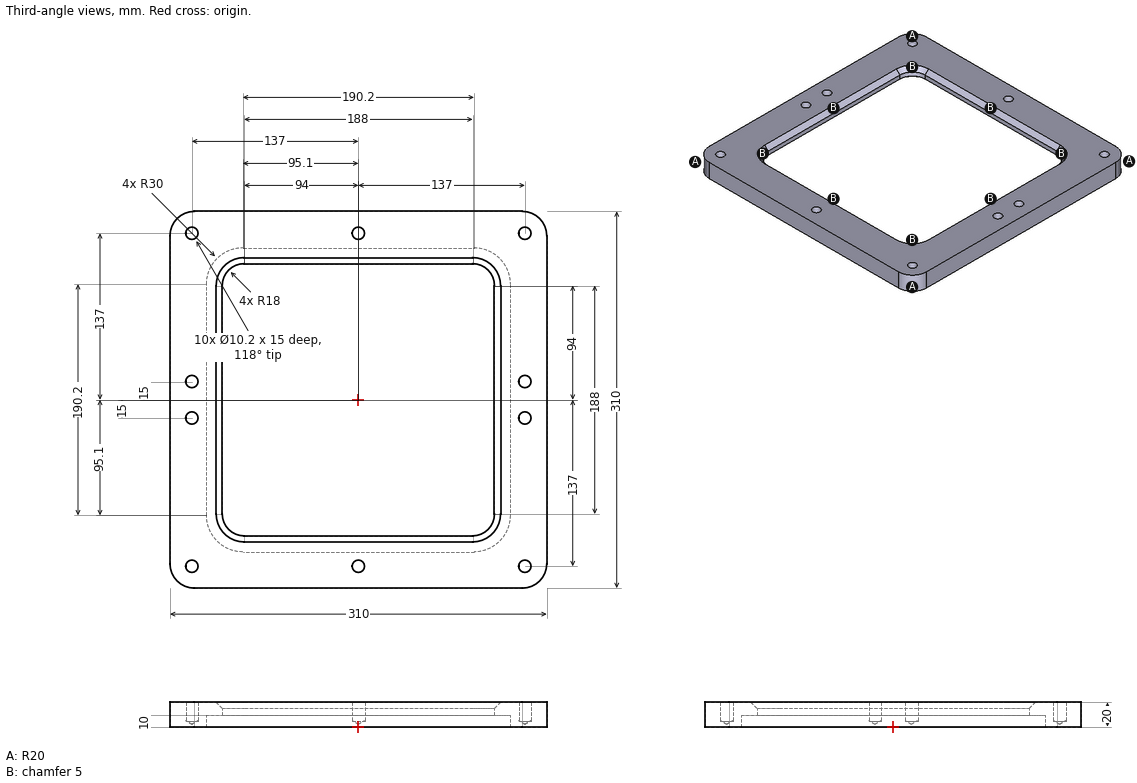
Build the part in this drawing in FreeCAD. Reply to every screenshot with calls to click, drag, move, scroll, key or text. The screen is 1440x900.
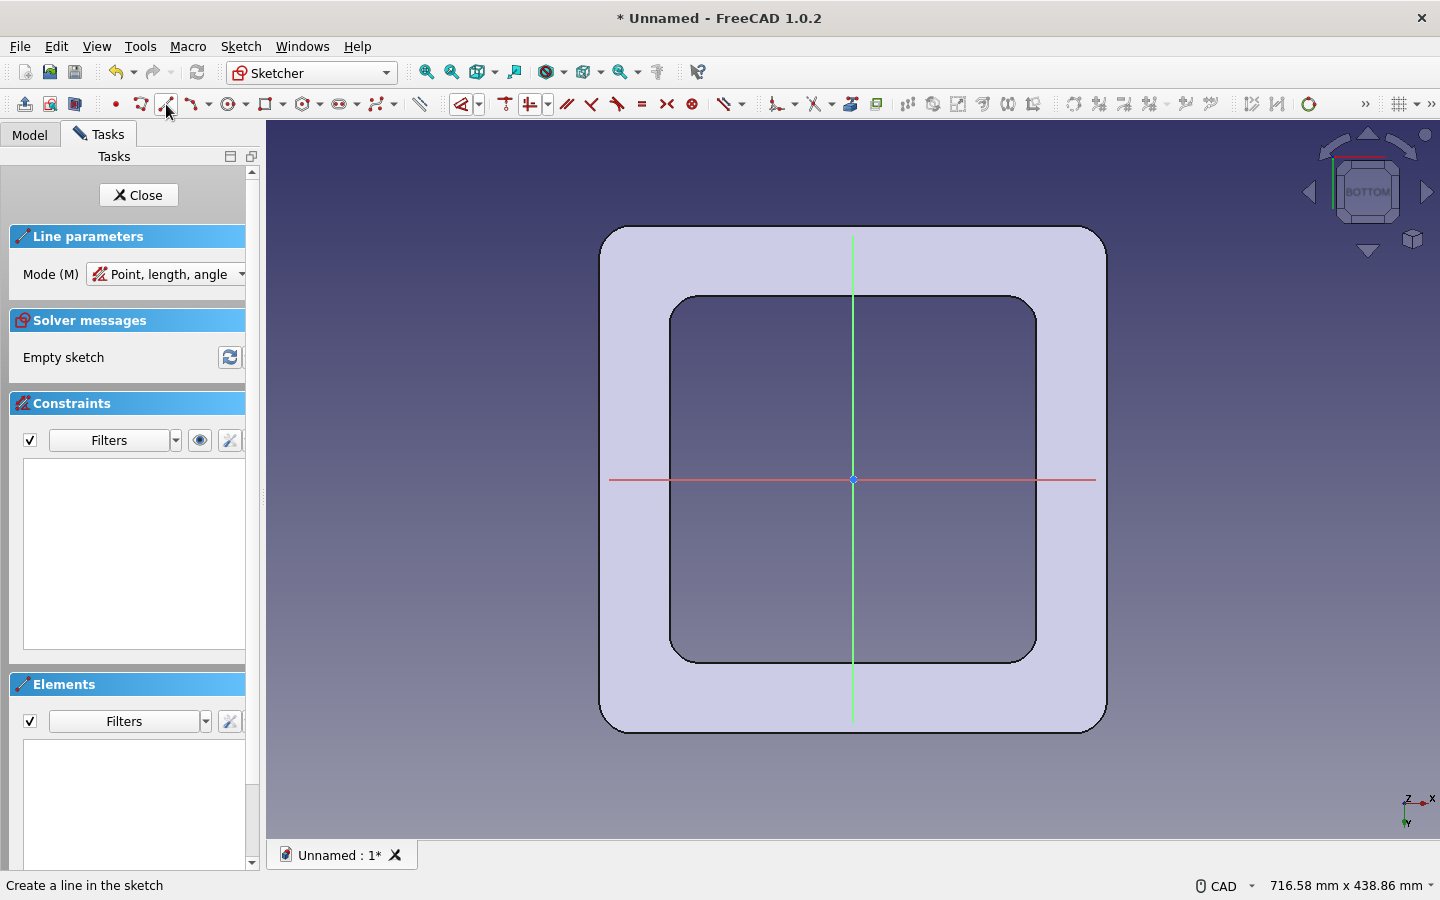
click(648, 324)
click(648, 635)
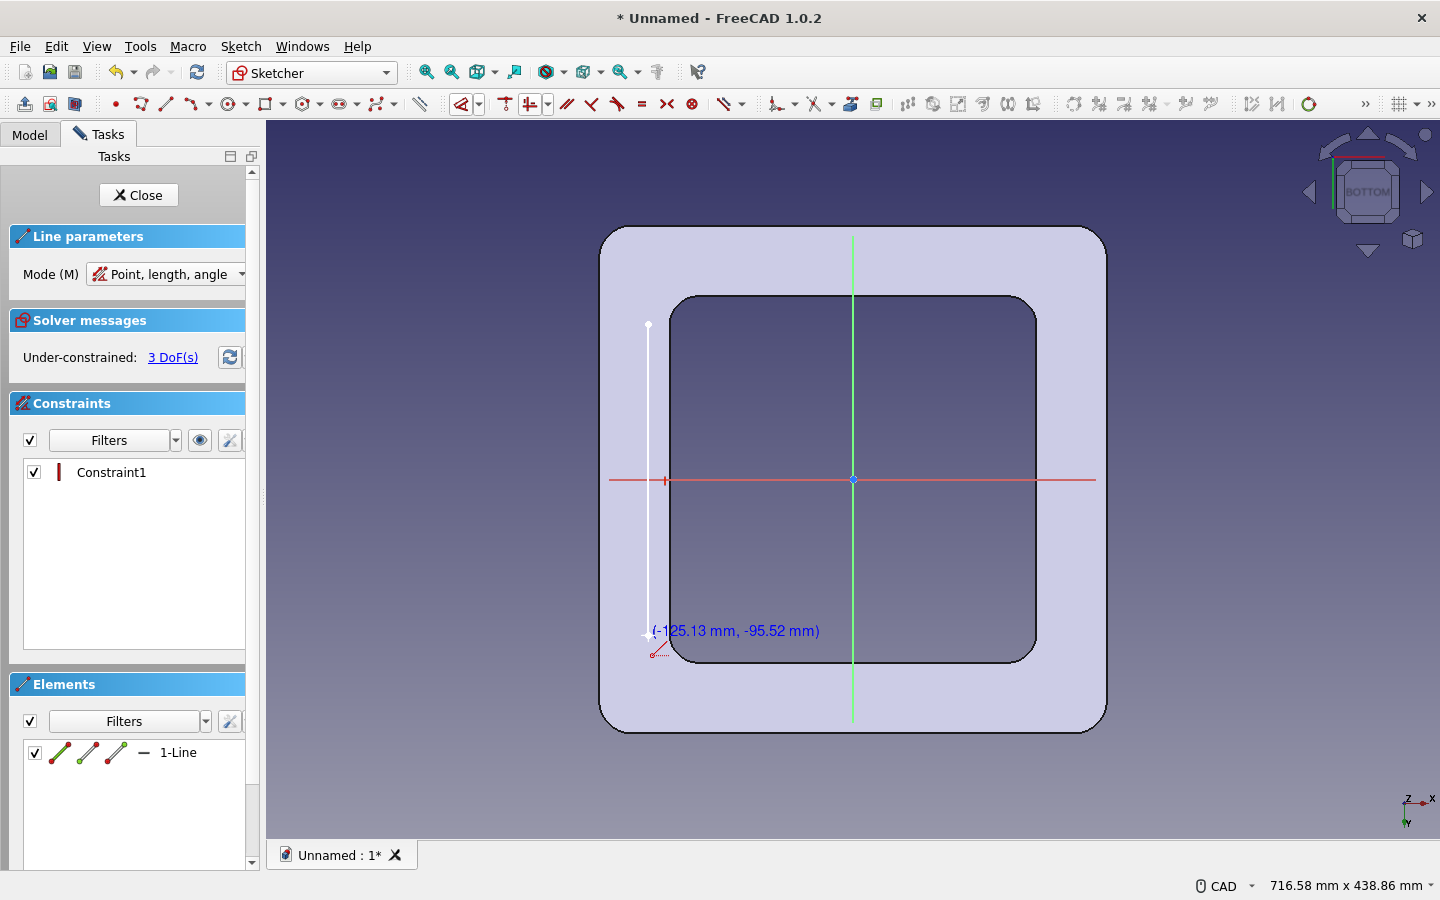
click(697, 684)
click(1009, 684)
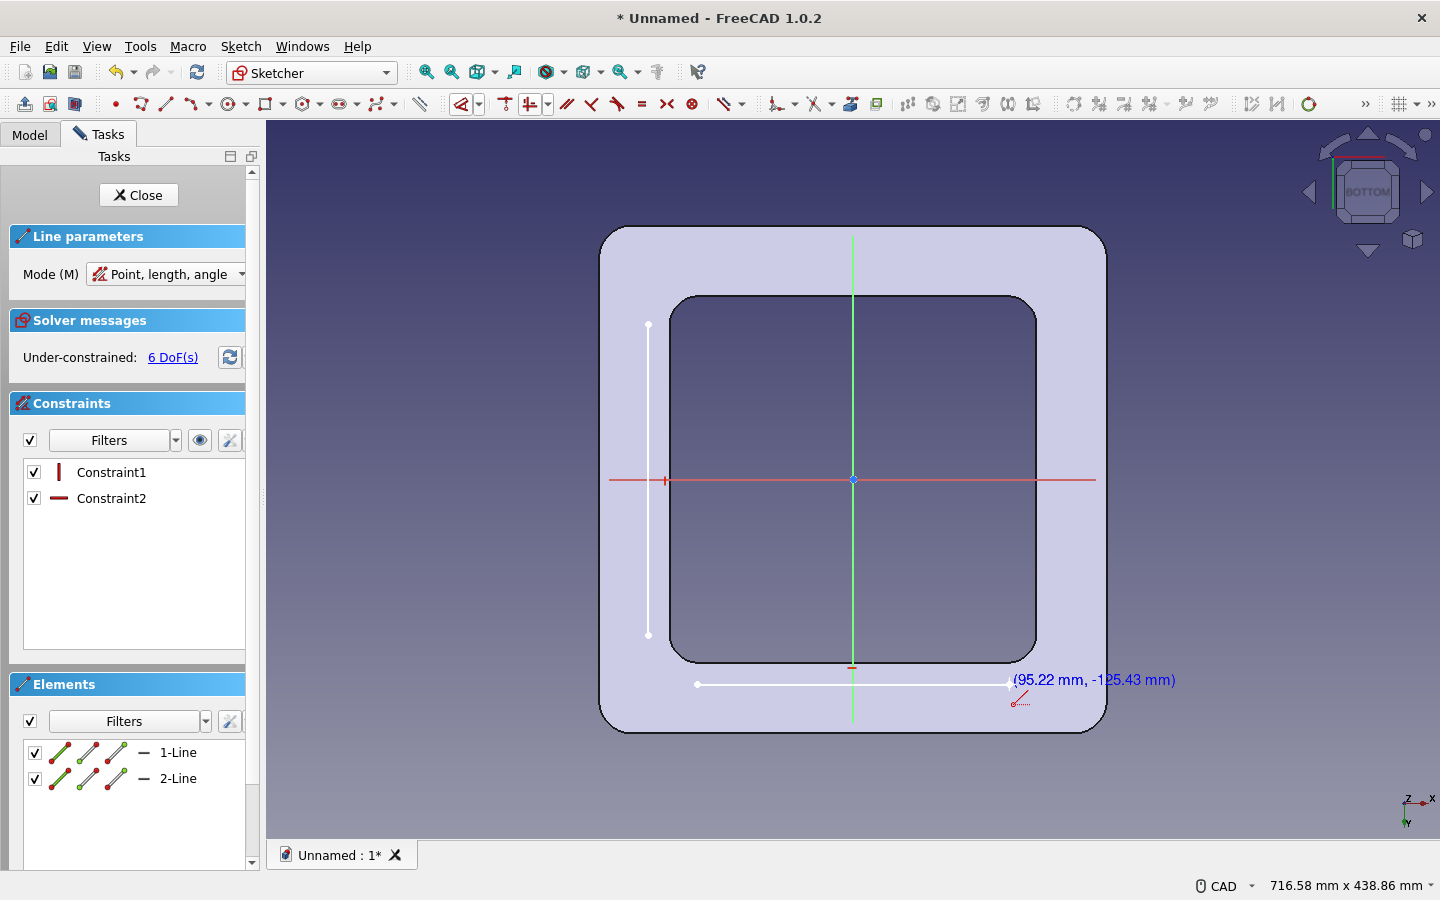
click(1058, 635)
click(1058, 324)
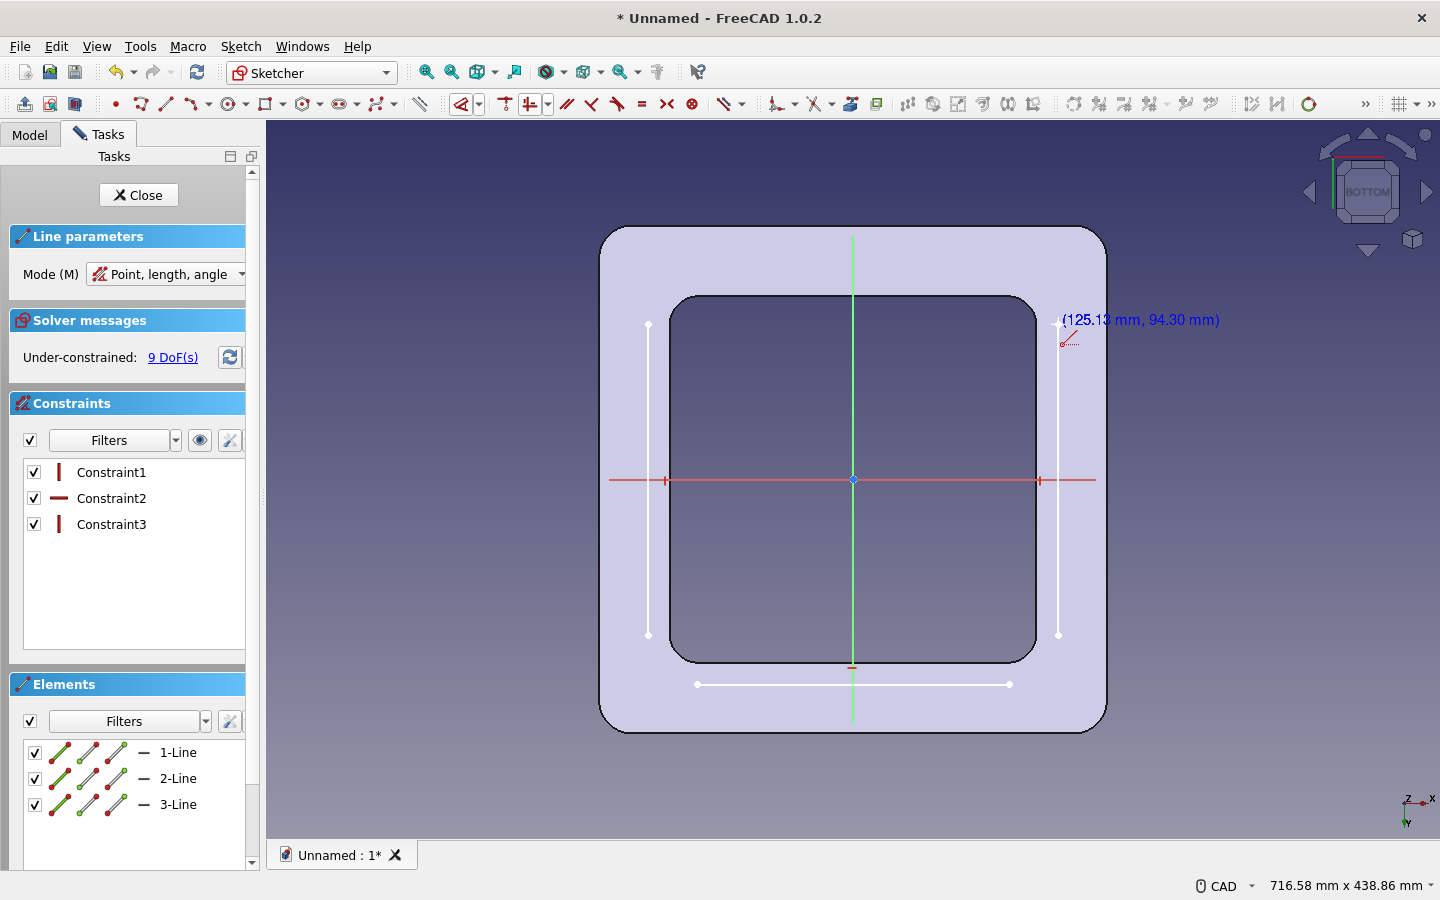
click(1009, 275)
click(697, 275)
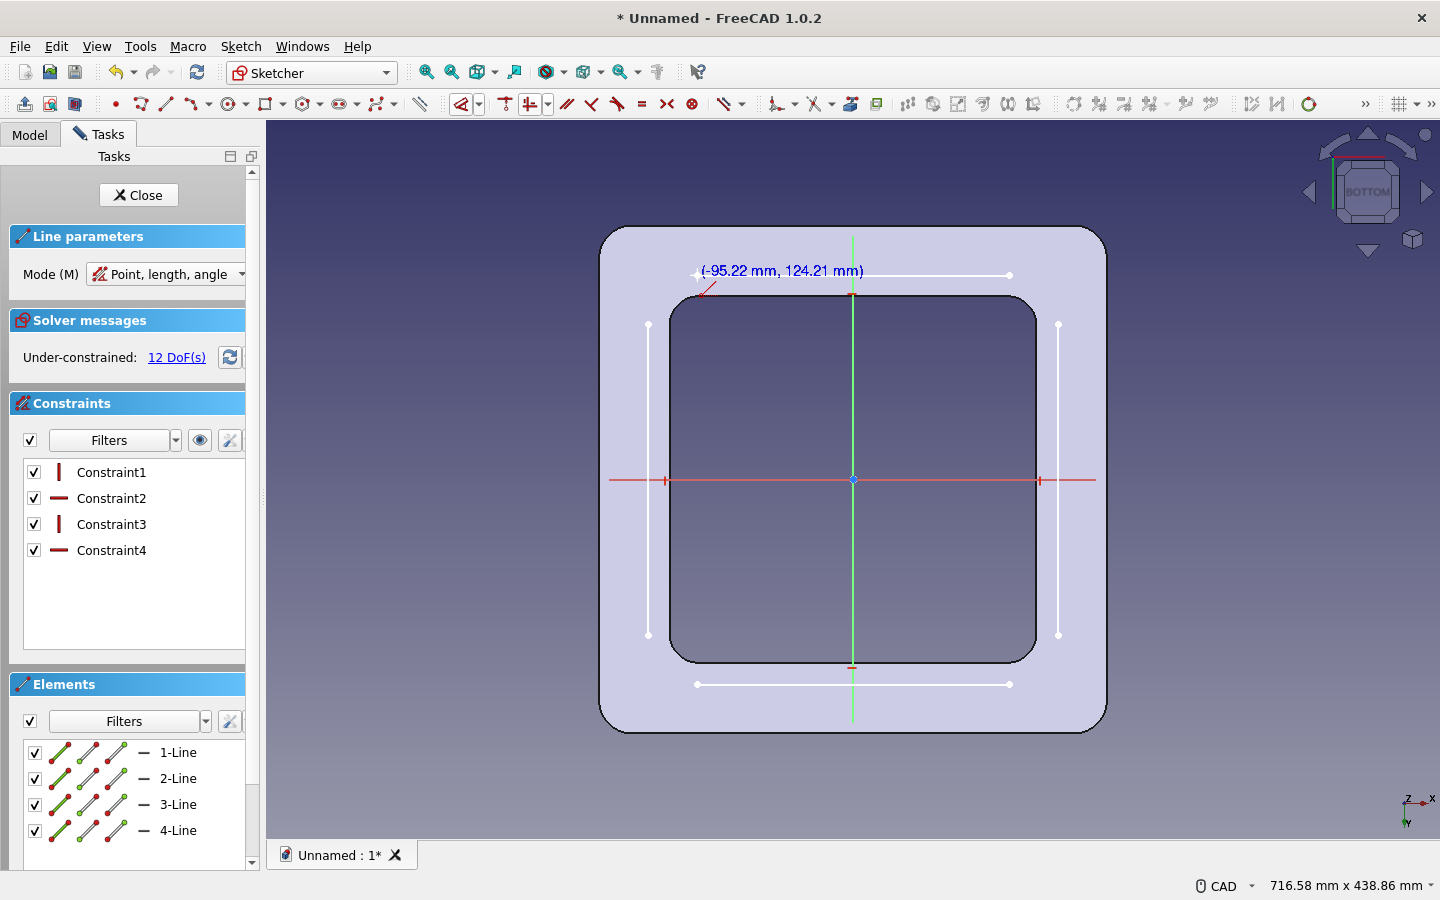
click(190, 104)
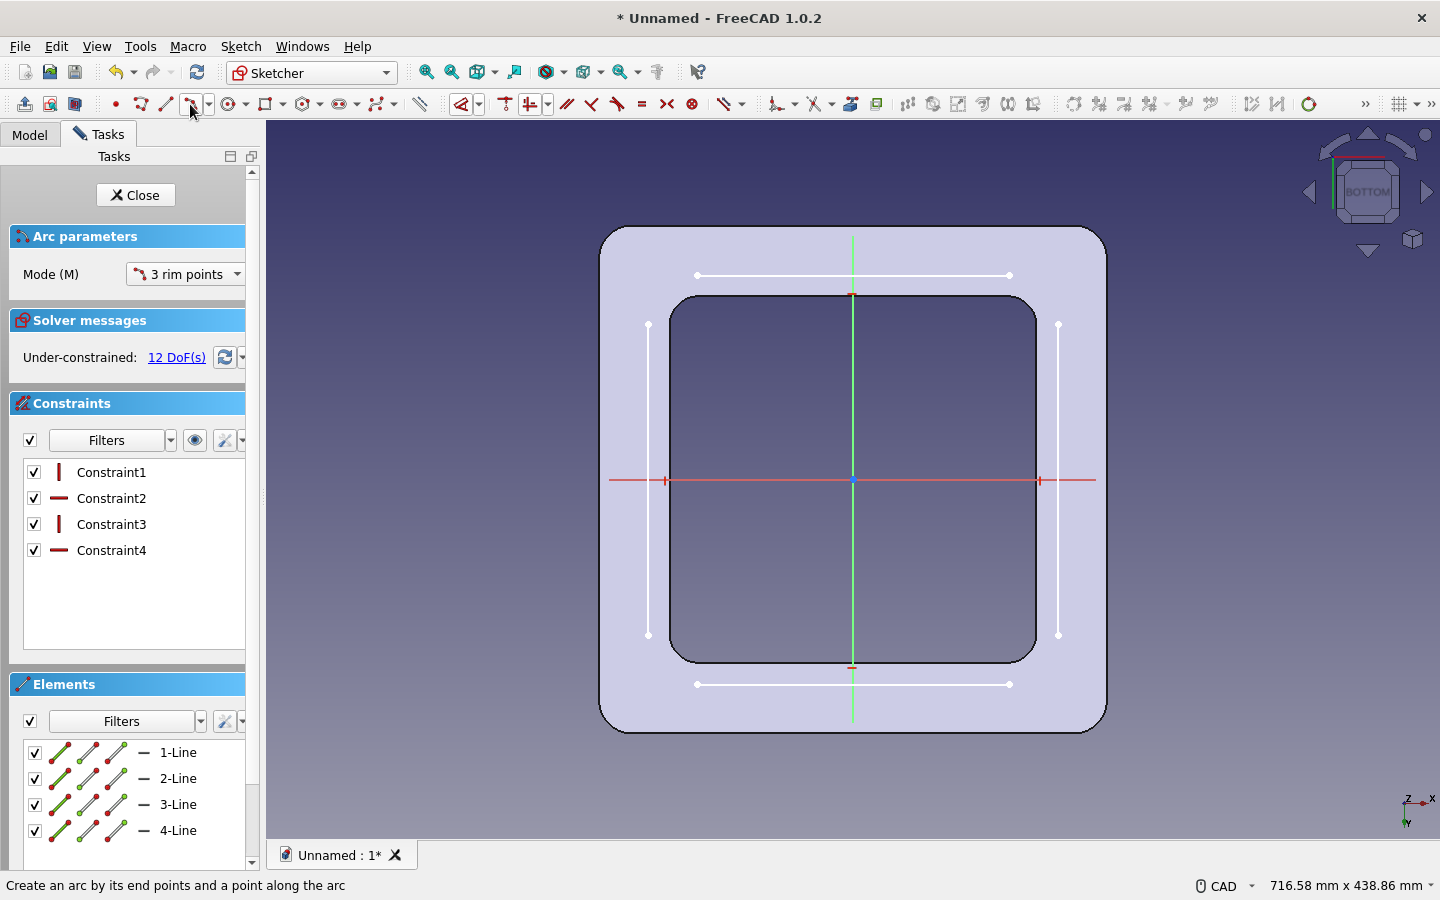
click(648, 636)
click(697, 685)
click(662, 670)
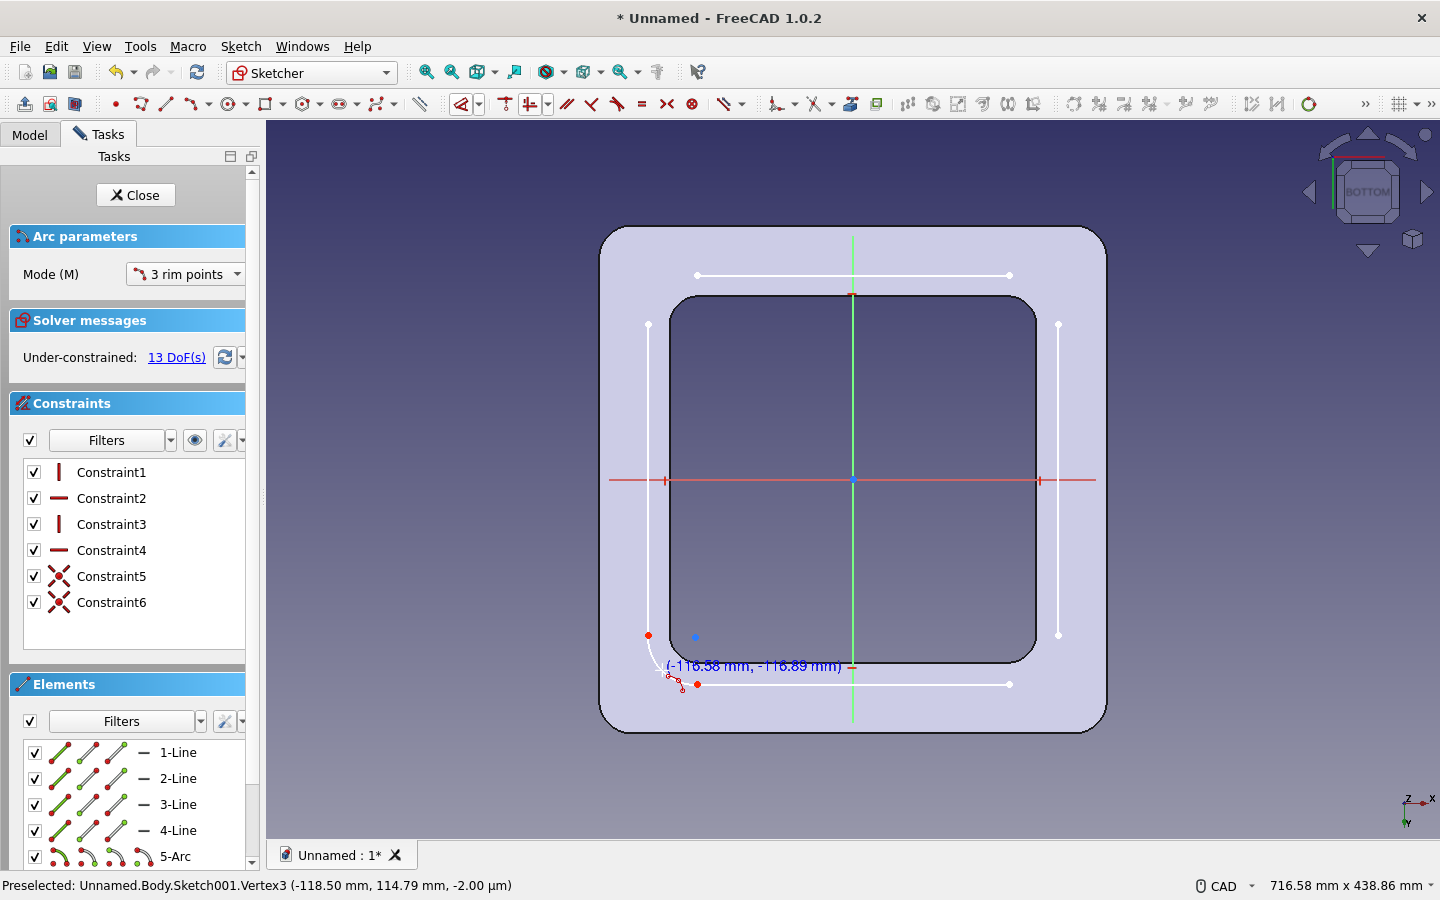
click(1009, 685)
click(1058, 636)
click(1044, 670)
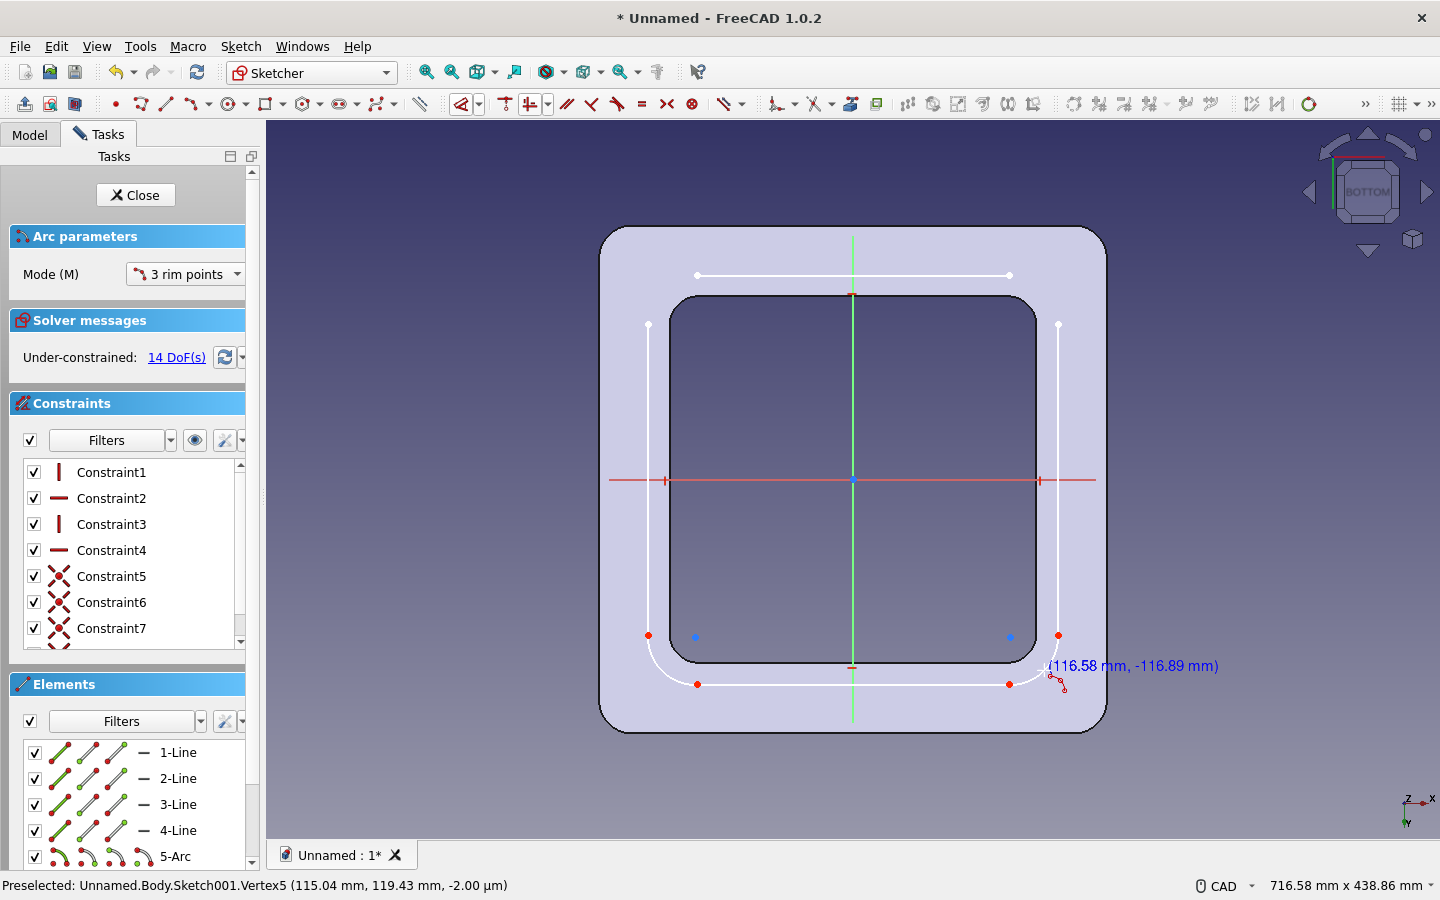
click(1058, 325)
click(1009, 276)
click(1044, 289)